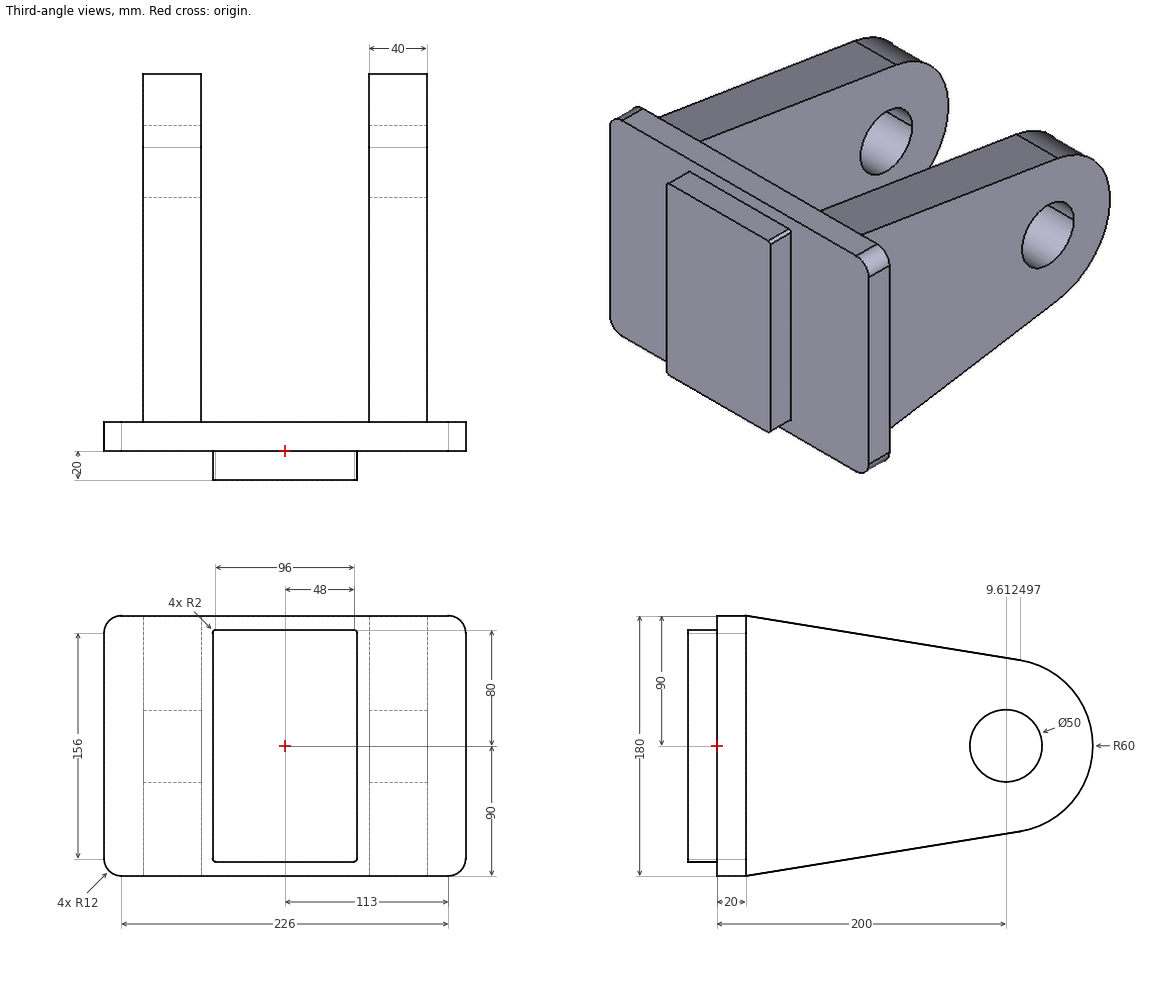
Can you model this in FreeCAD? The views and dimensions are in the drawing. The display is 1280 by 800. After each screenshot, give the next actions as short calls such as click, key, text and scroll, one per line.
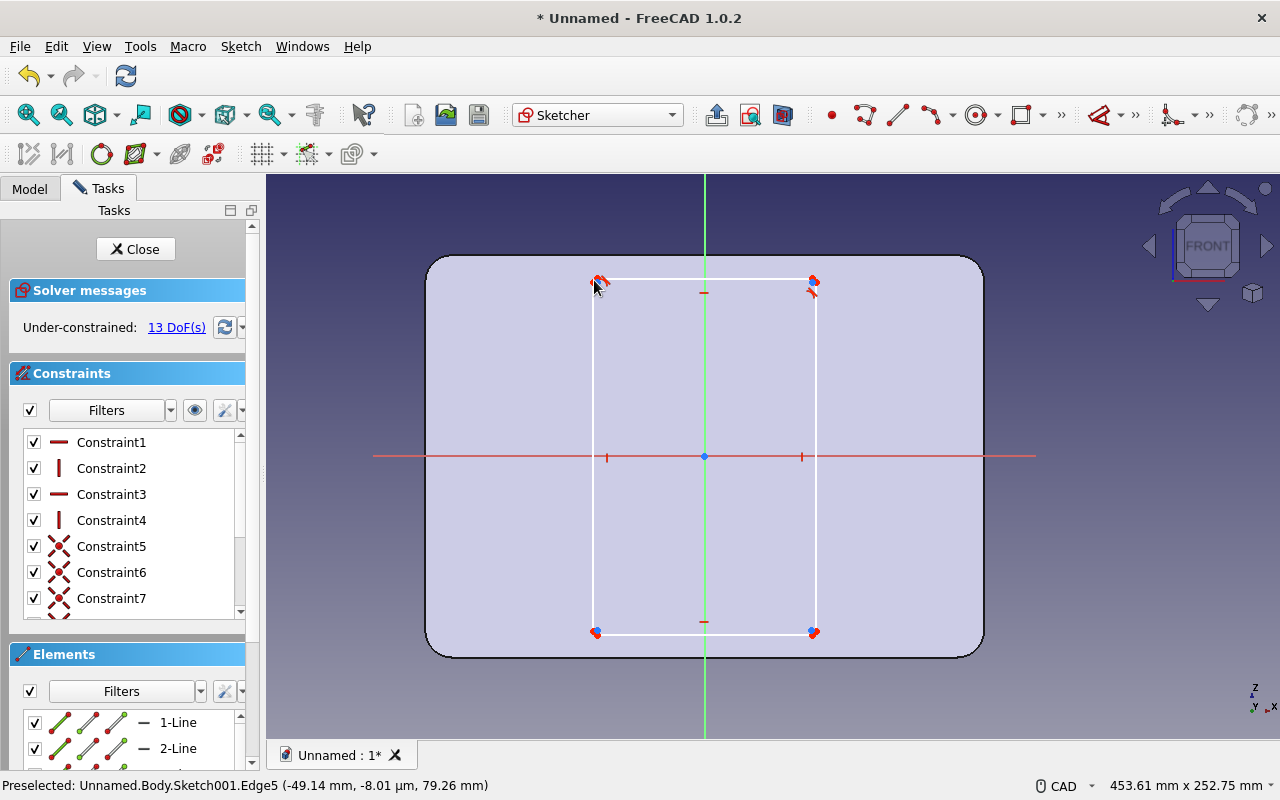
click(593, 352)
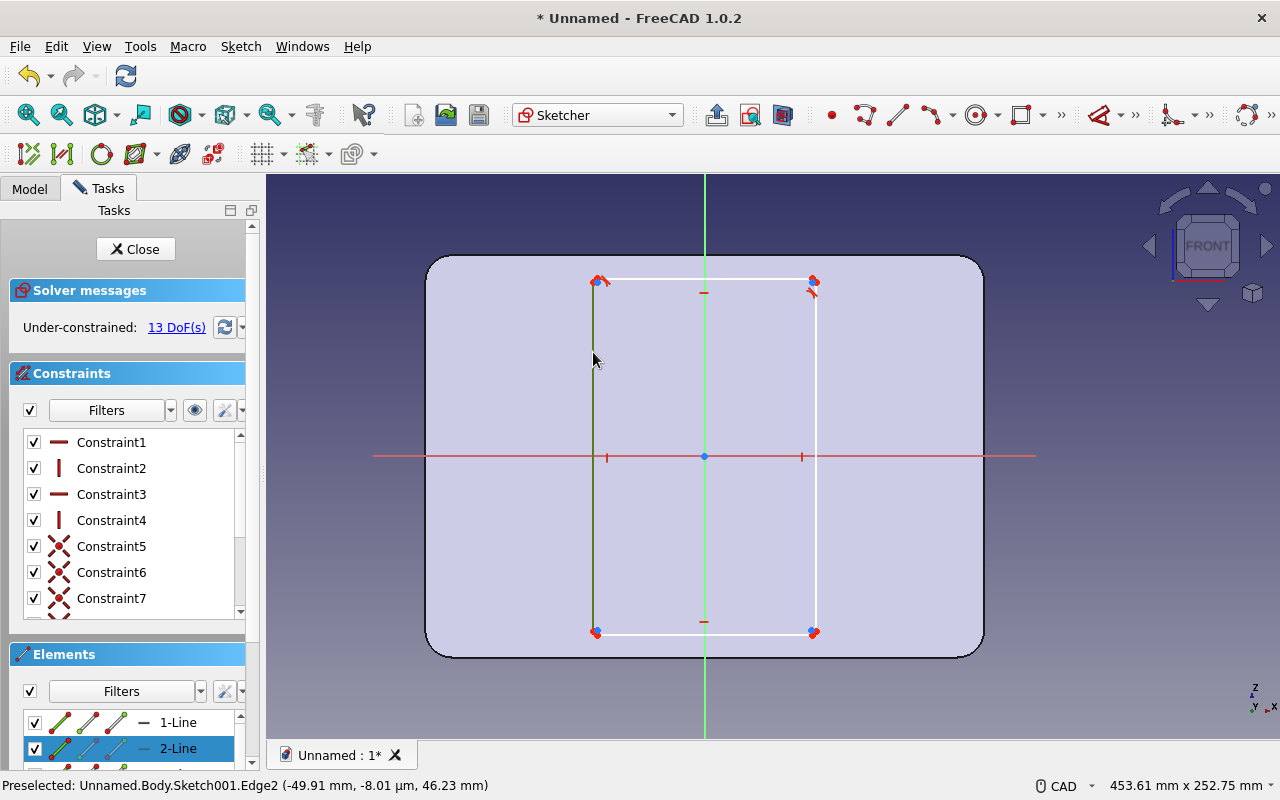
scroll(595, 634, up, 8)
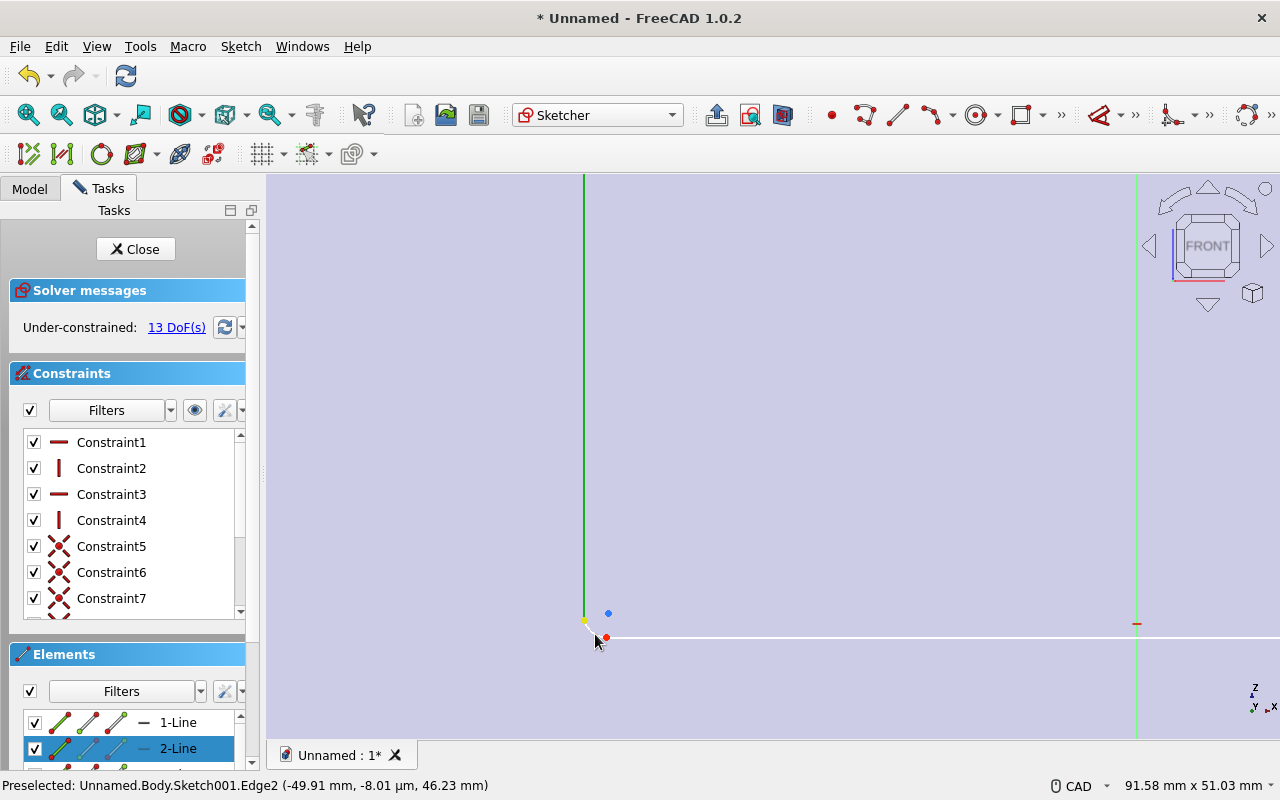
click(593, 633)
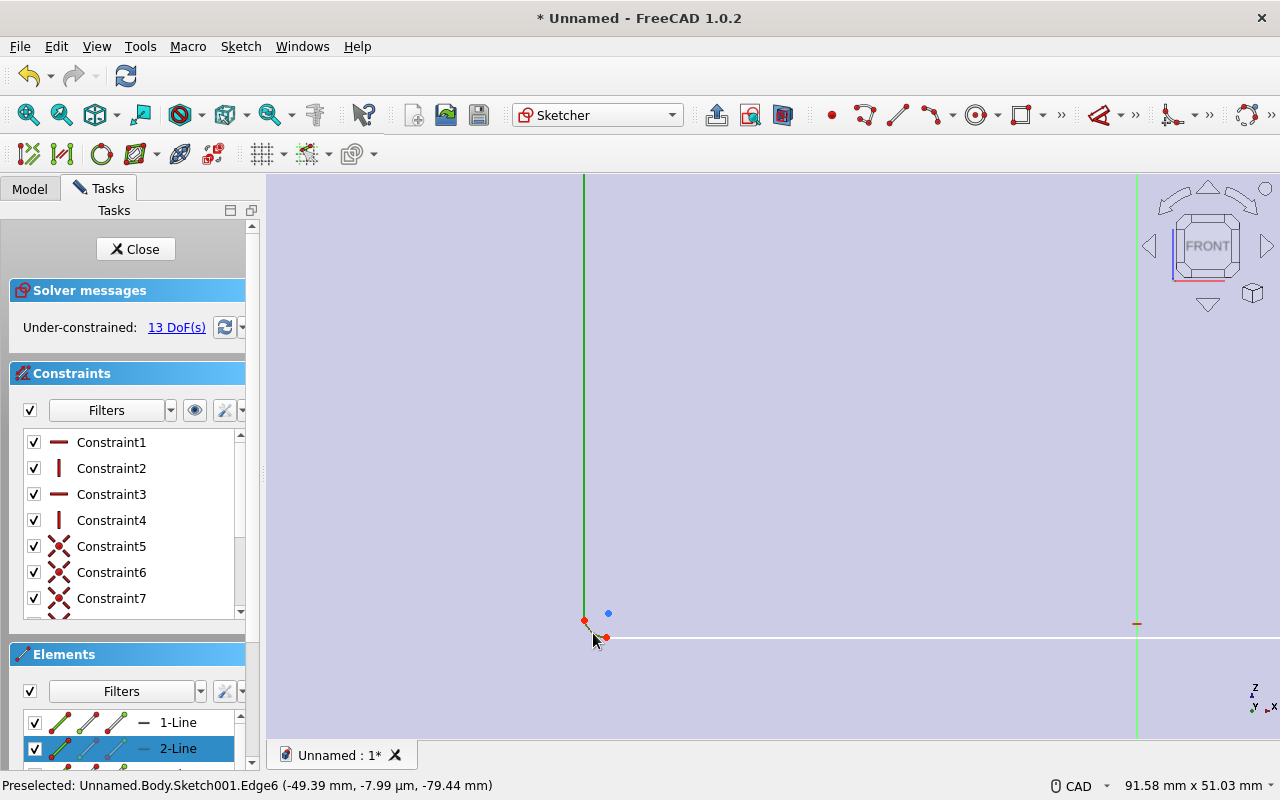
key(t)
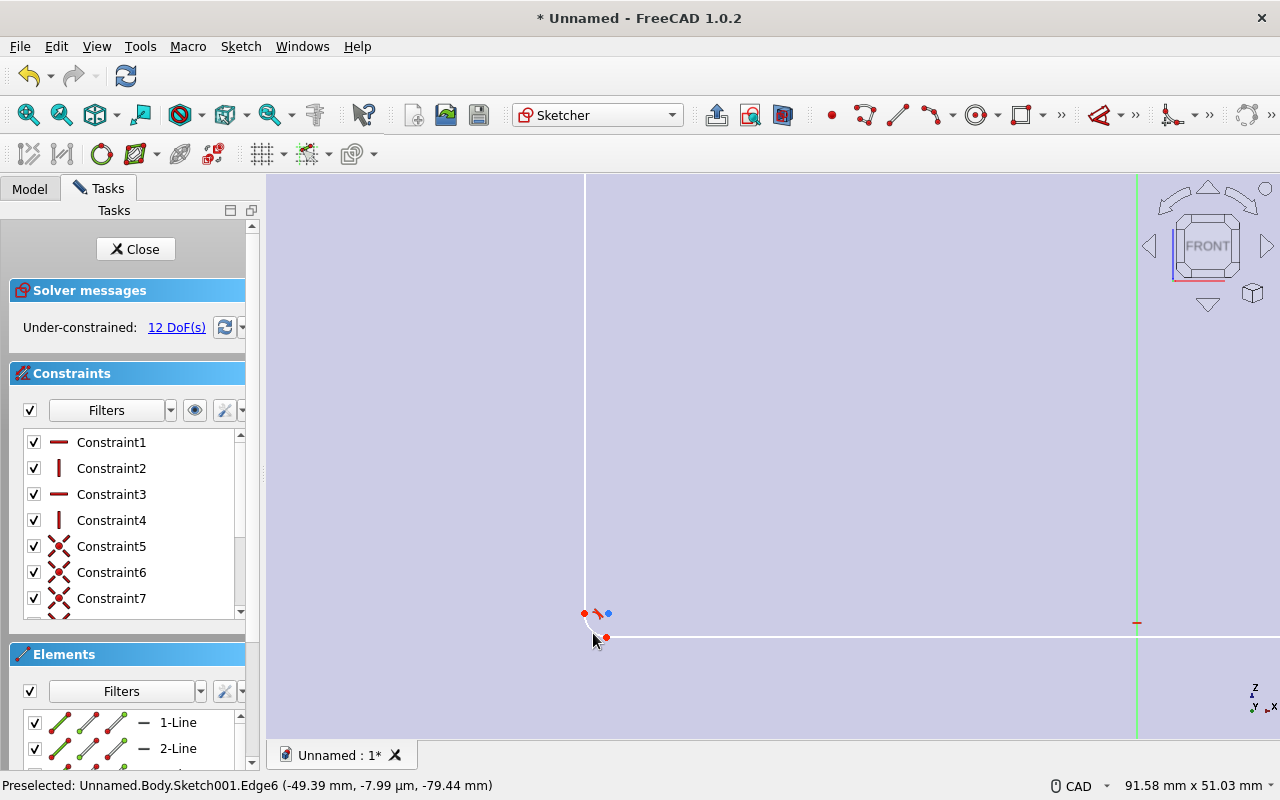
scroll(595, 635, down, 8)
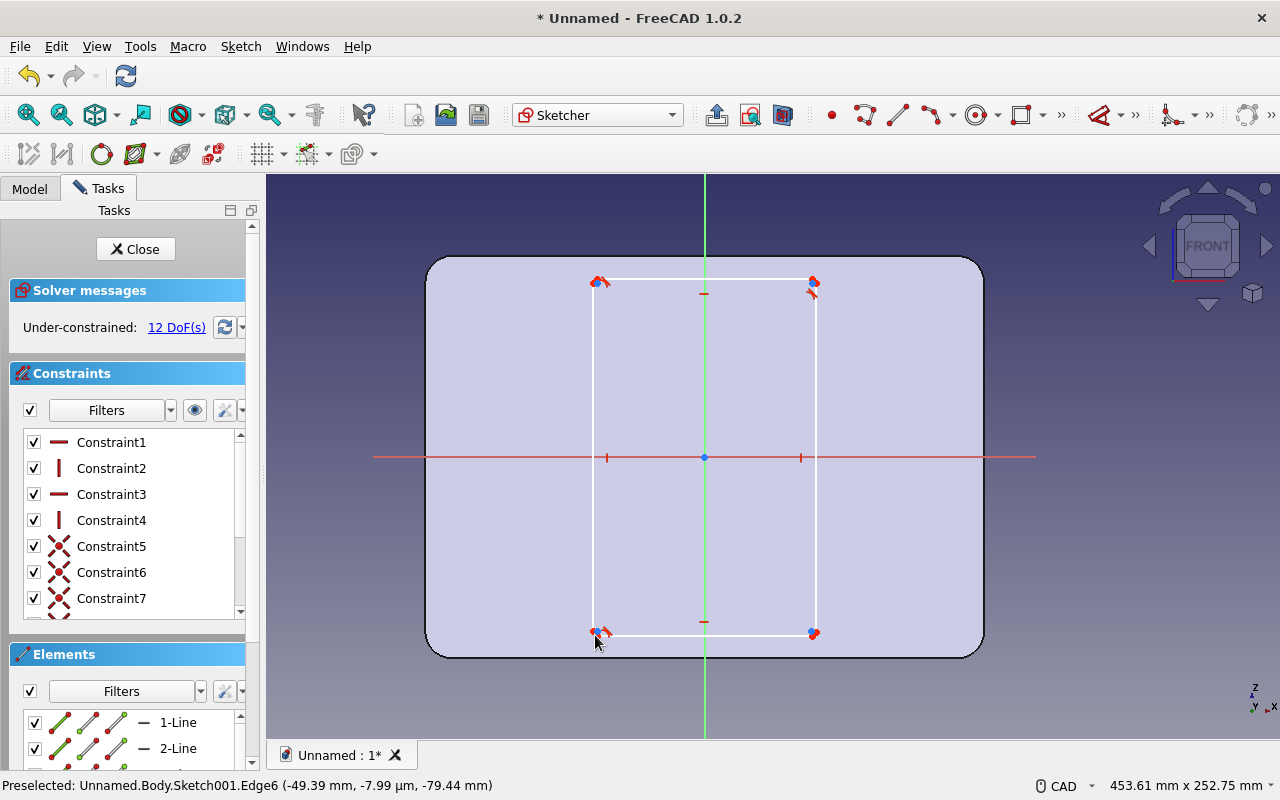
click(662, 636)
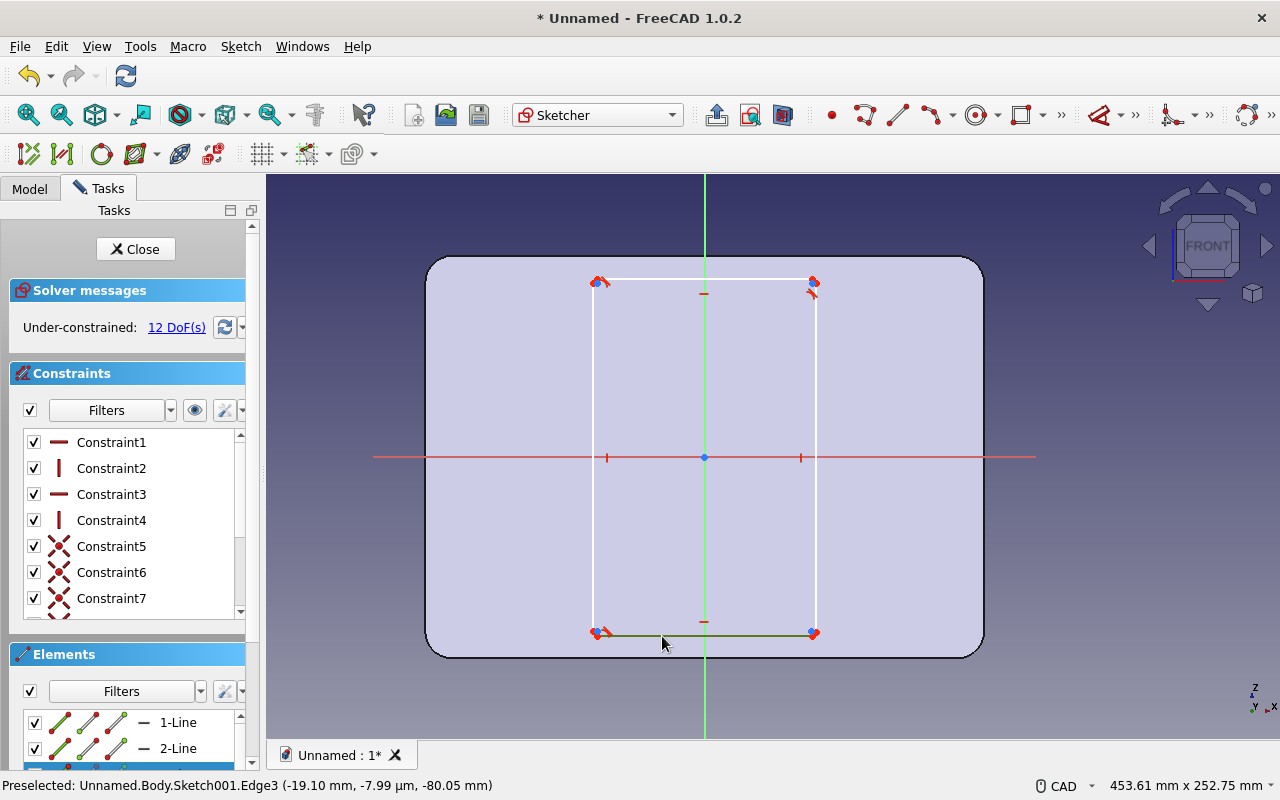
scroll(594, 635, up, 7)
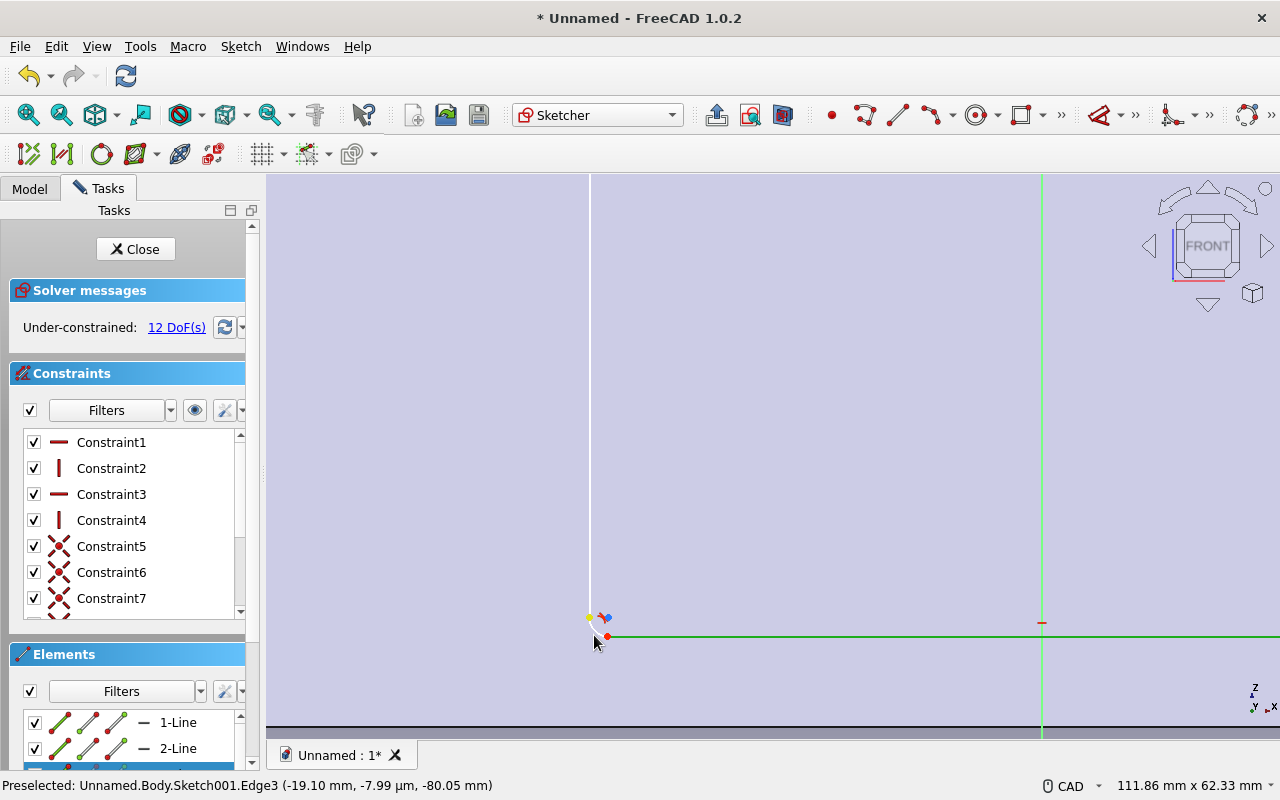
click(595, 631)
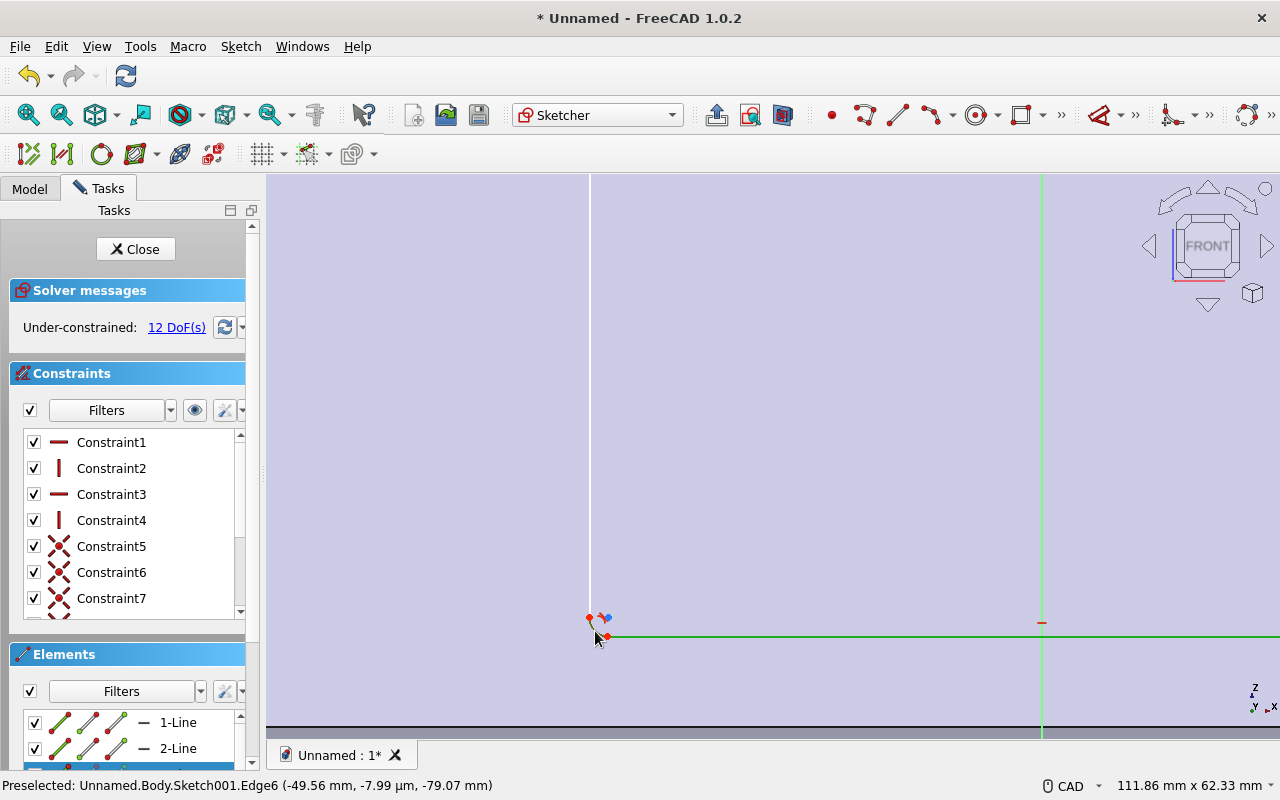
key(t)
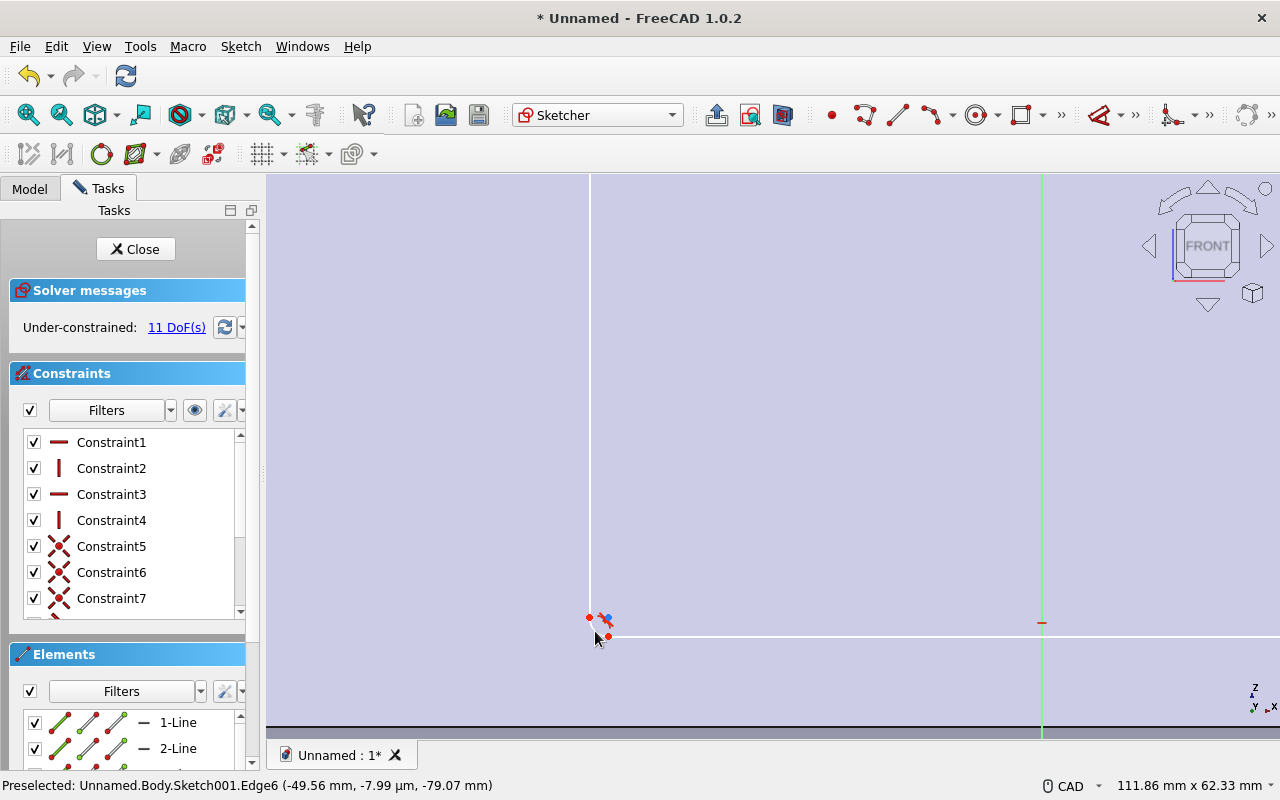
scroll(594, 635, down, 7)